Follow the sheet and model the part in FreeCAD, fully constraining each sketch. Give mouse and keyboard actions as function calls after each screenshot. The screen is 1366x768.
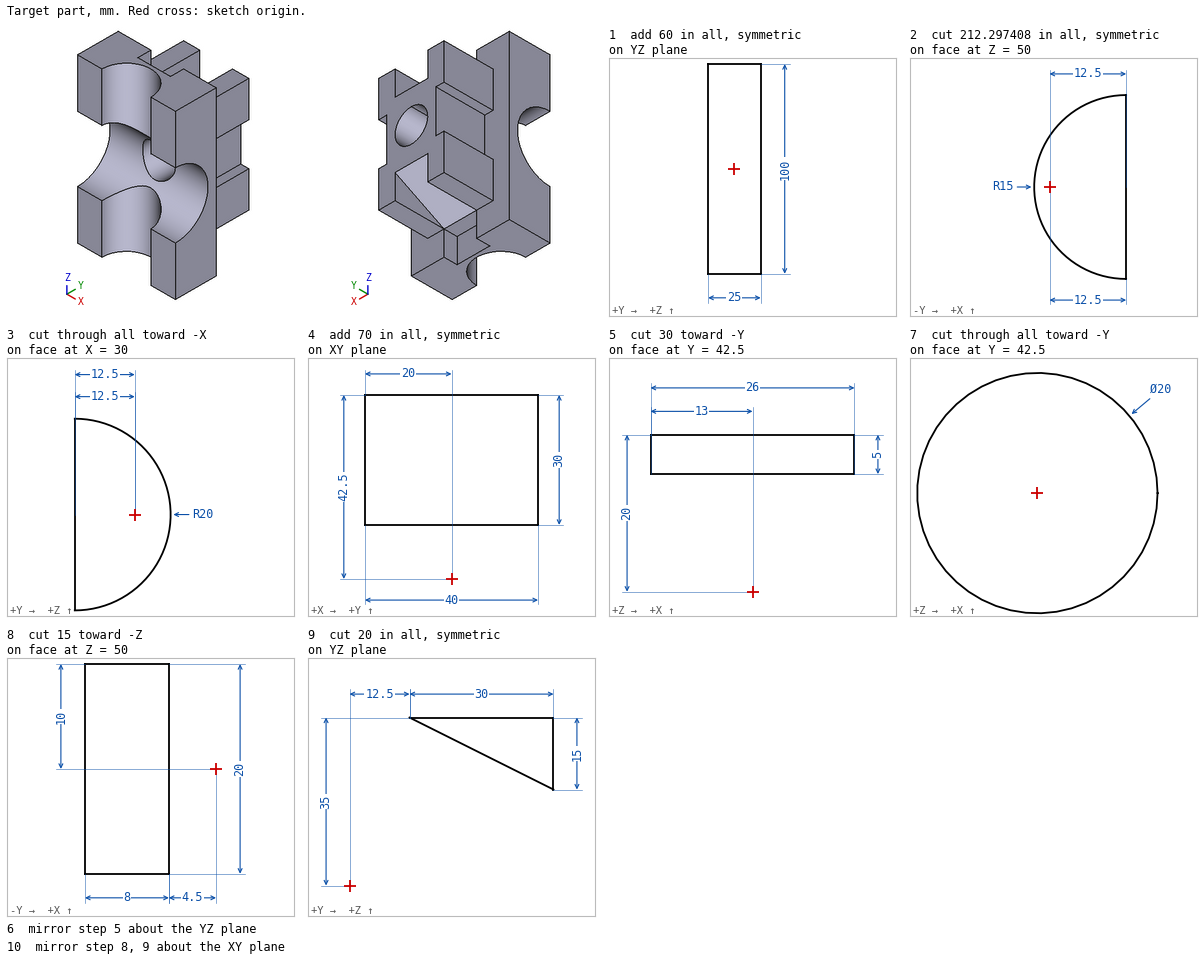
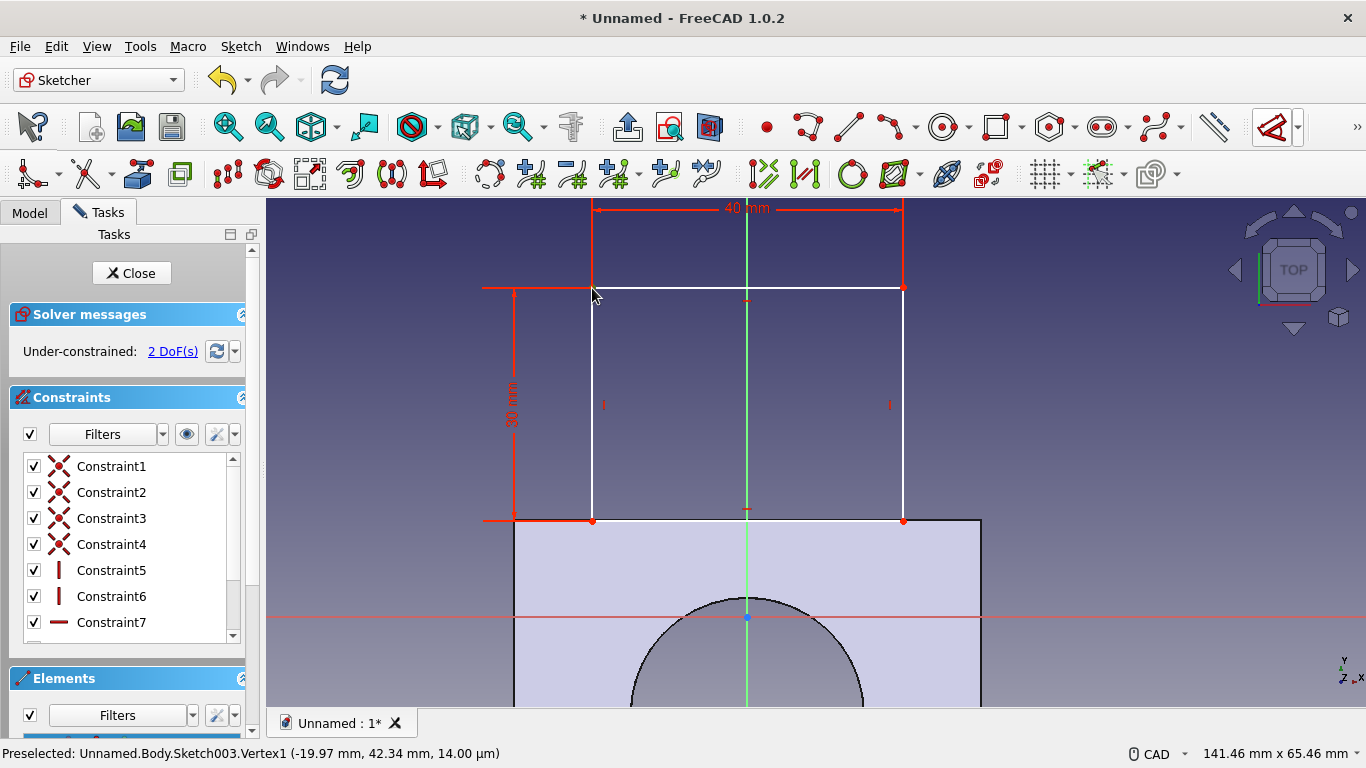
key(l)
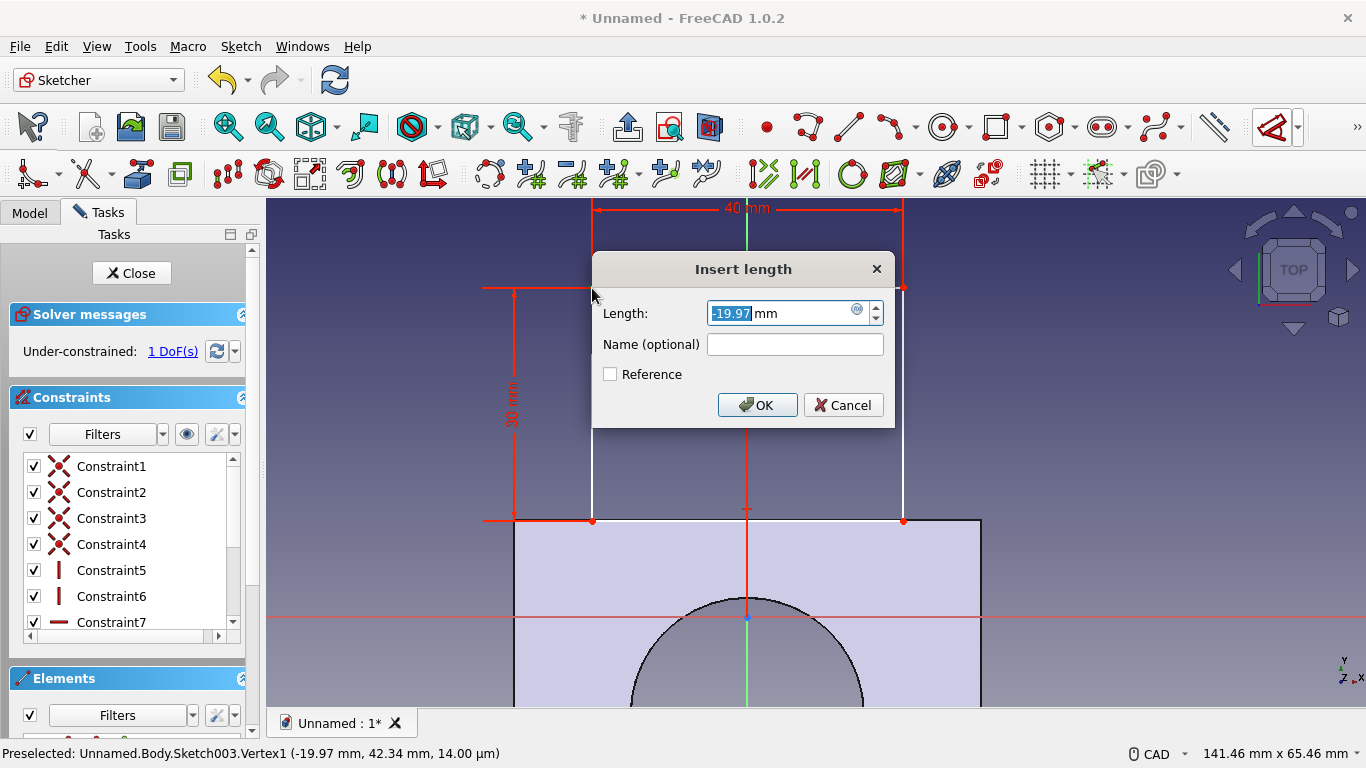
text(-20)
key(Return)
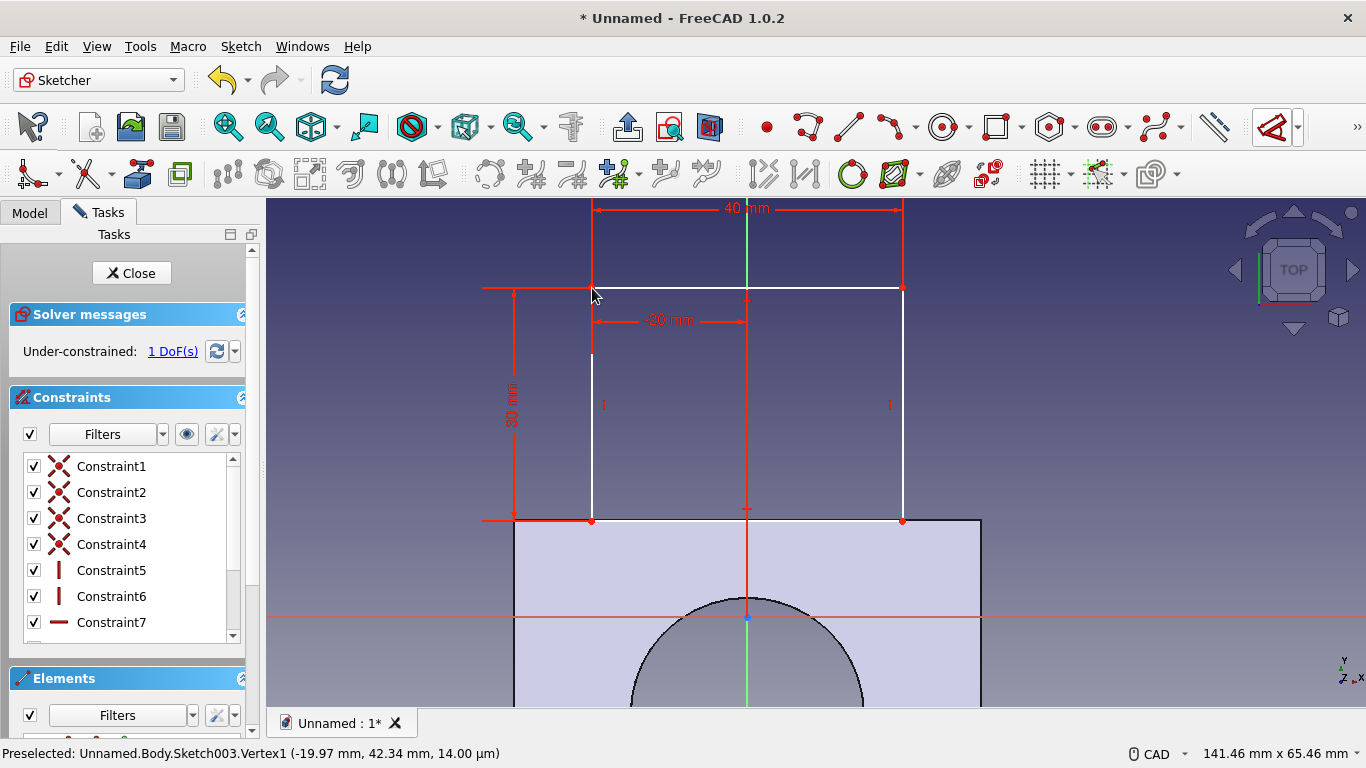
click(592, 288)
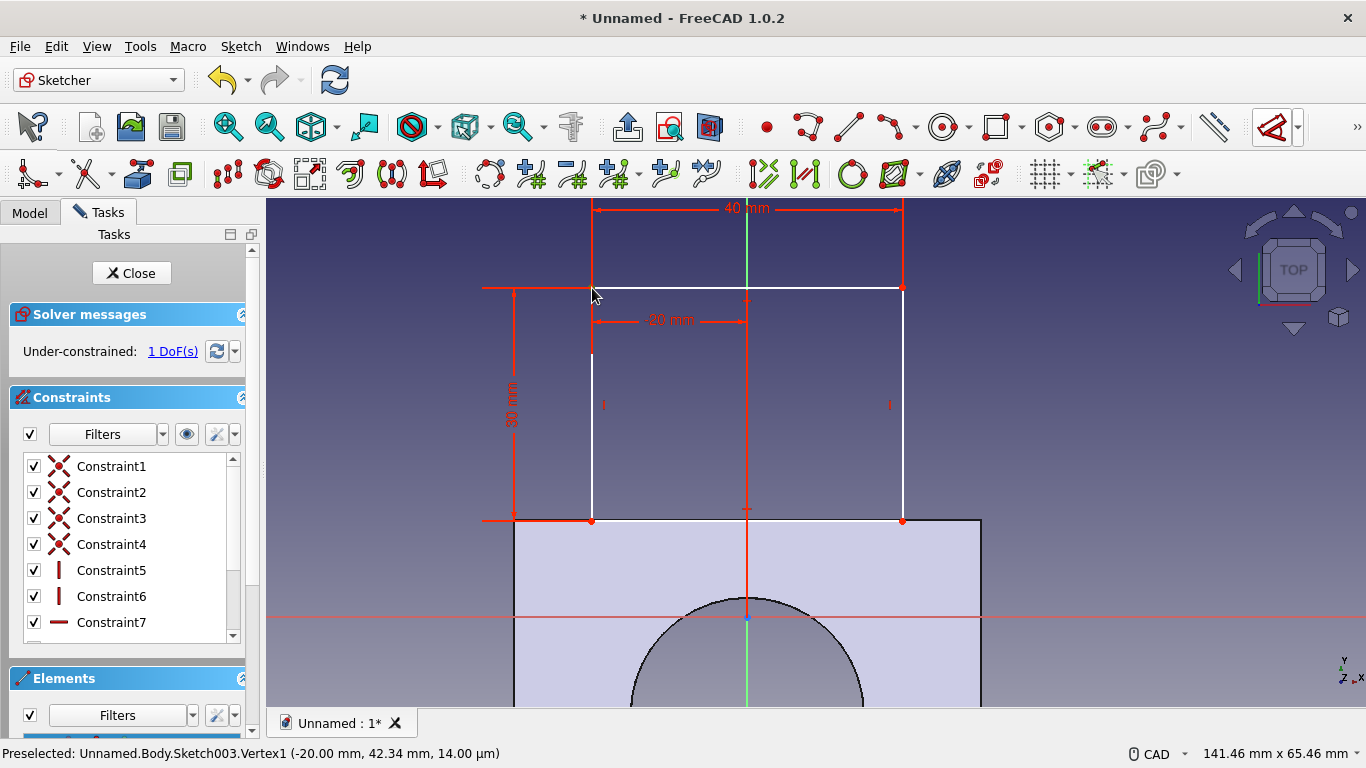
key(i)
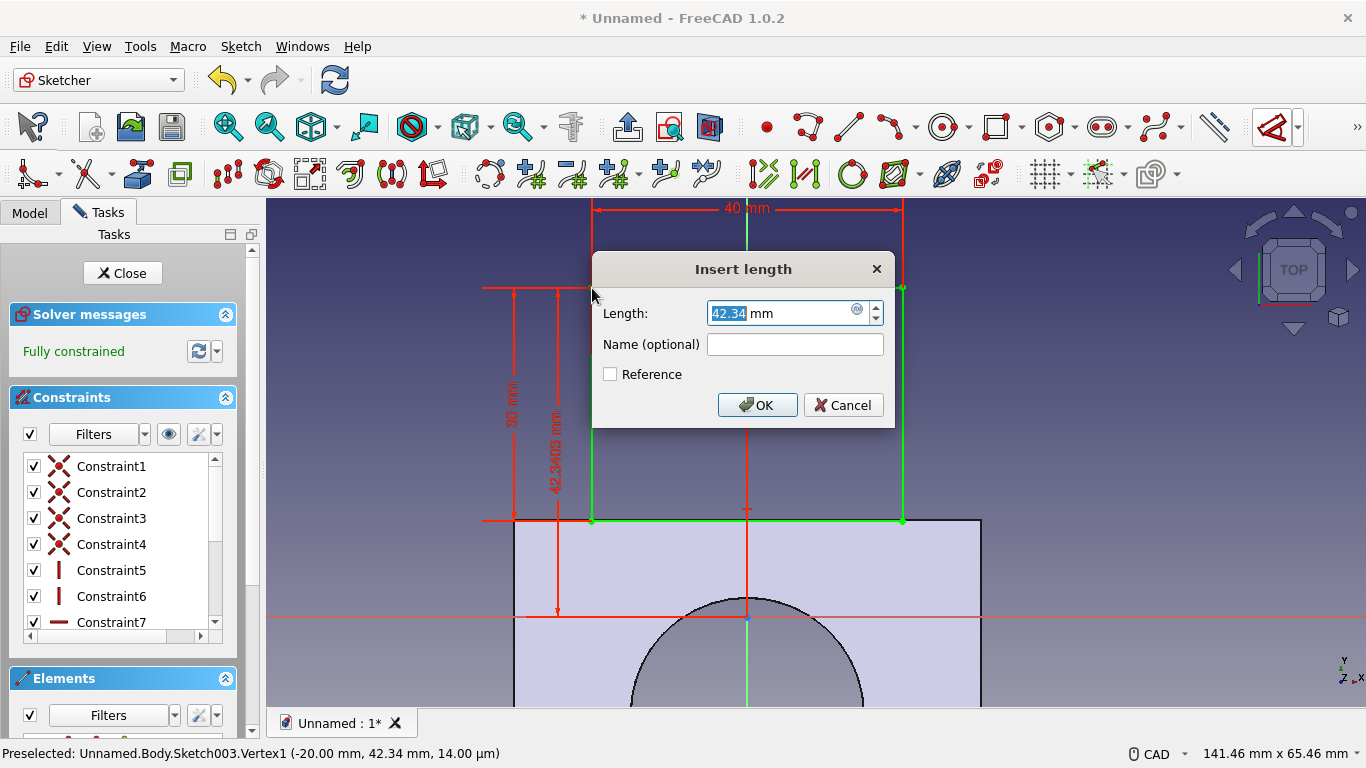
text(42.5)
key(Return)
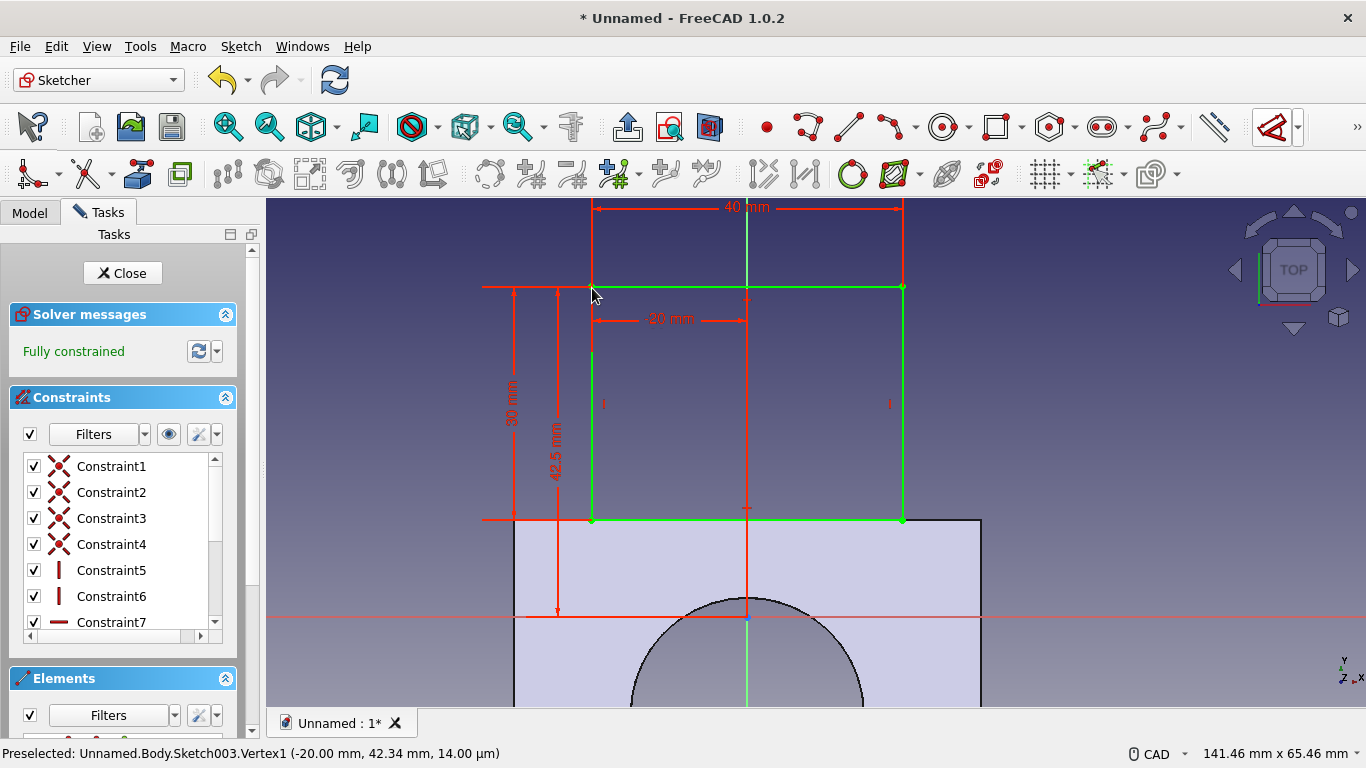
click(123, 273)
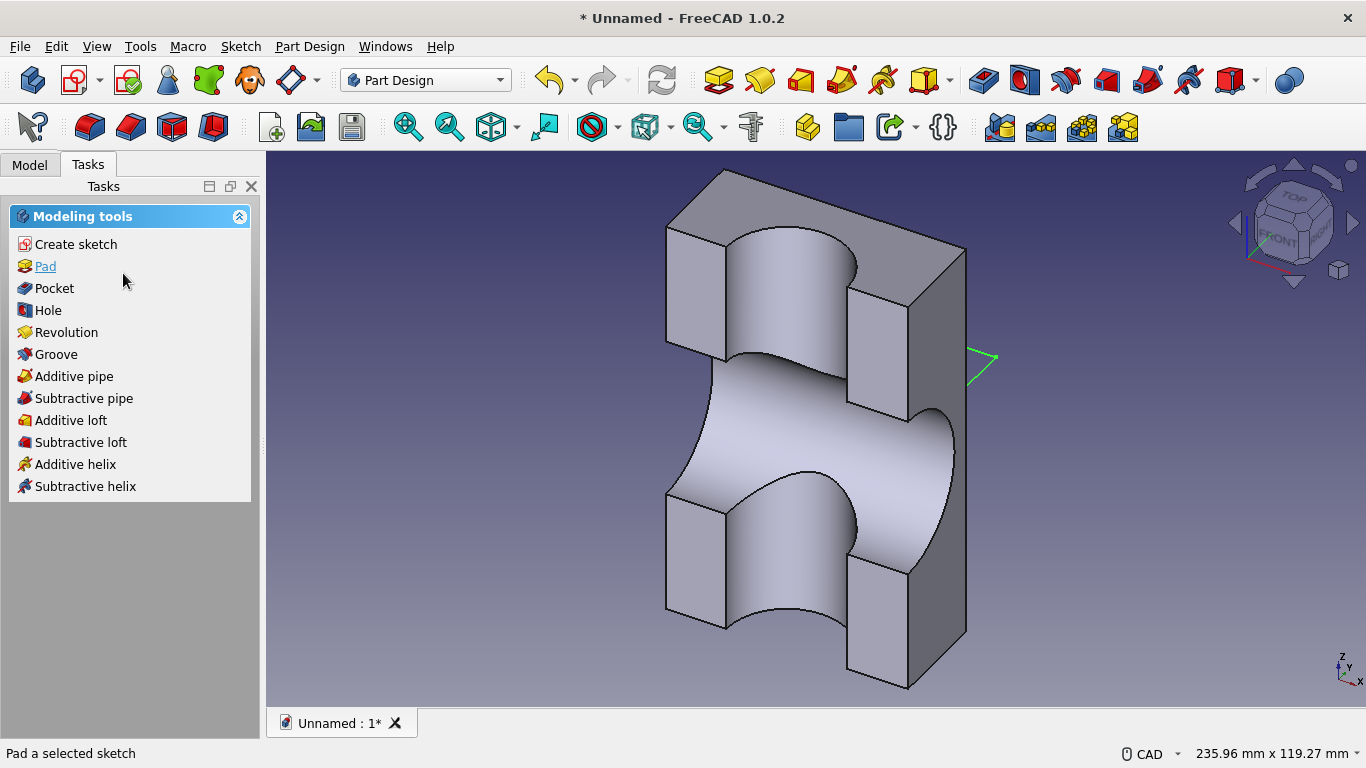
click(719, 80)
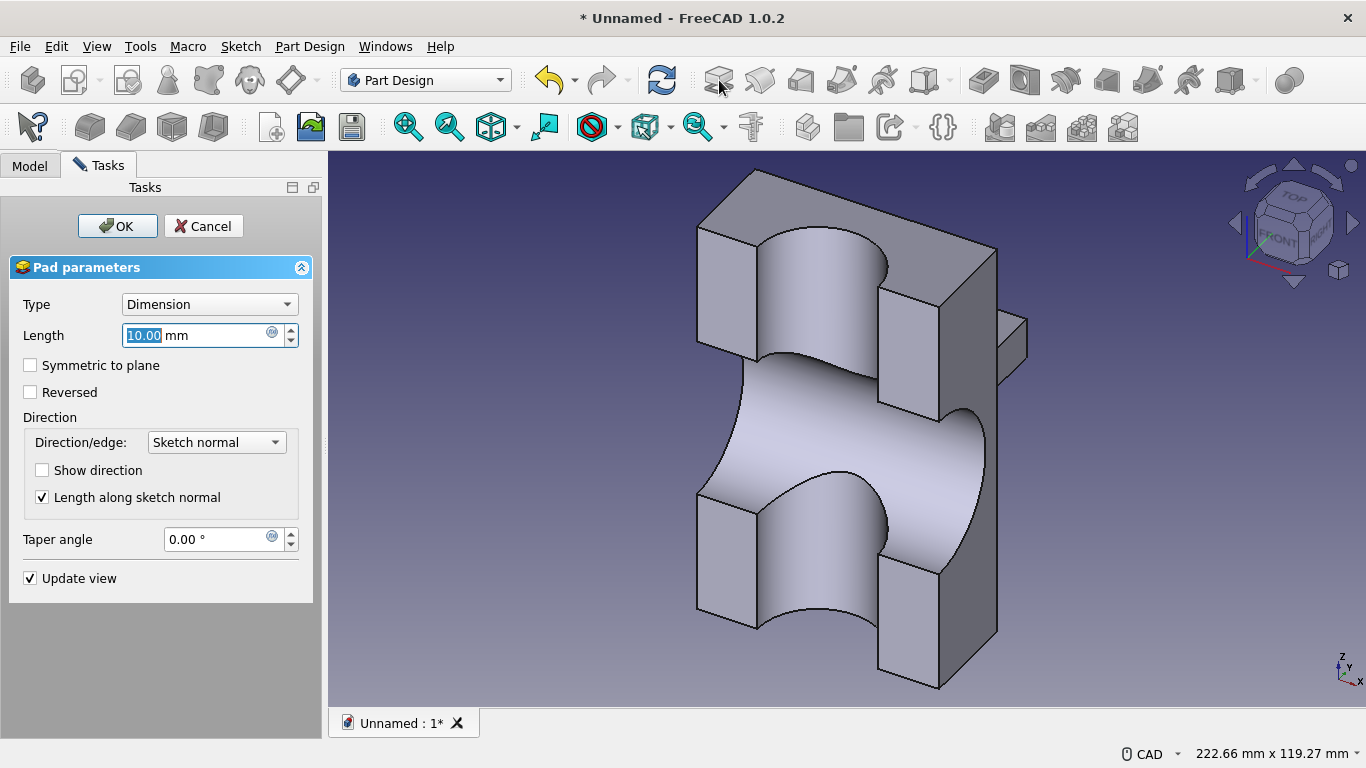
text(70)
key(Tab)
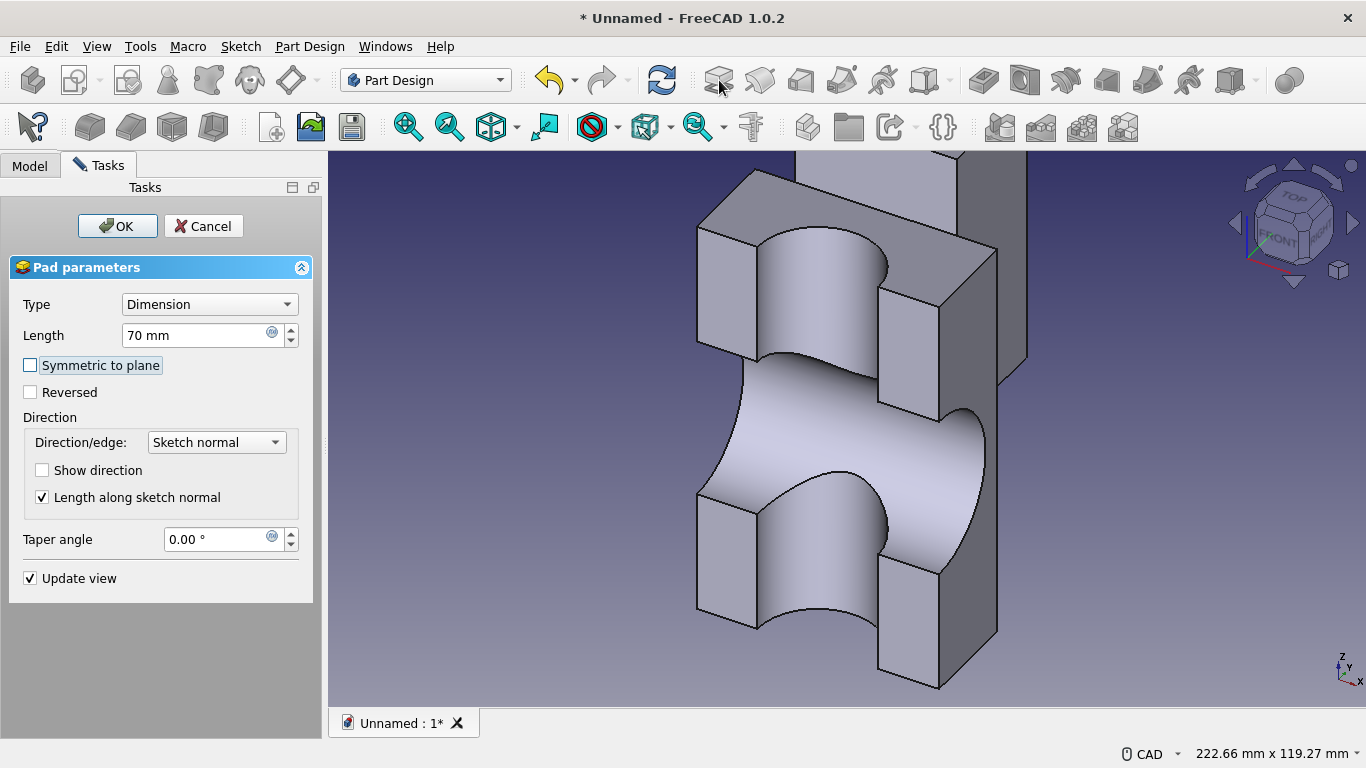
click(31, 365)